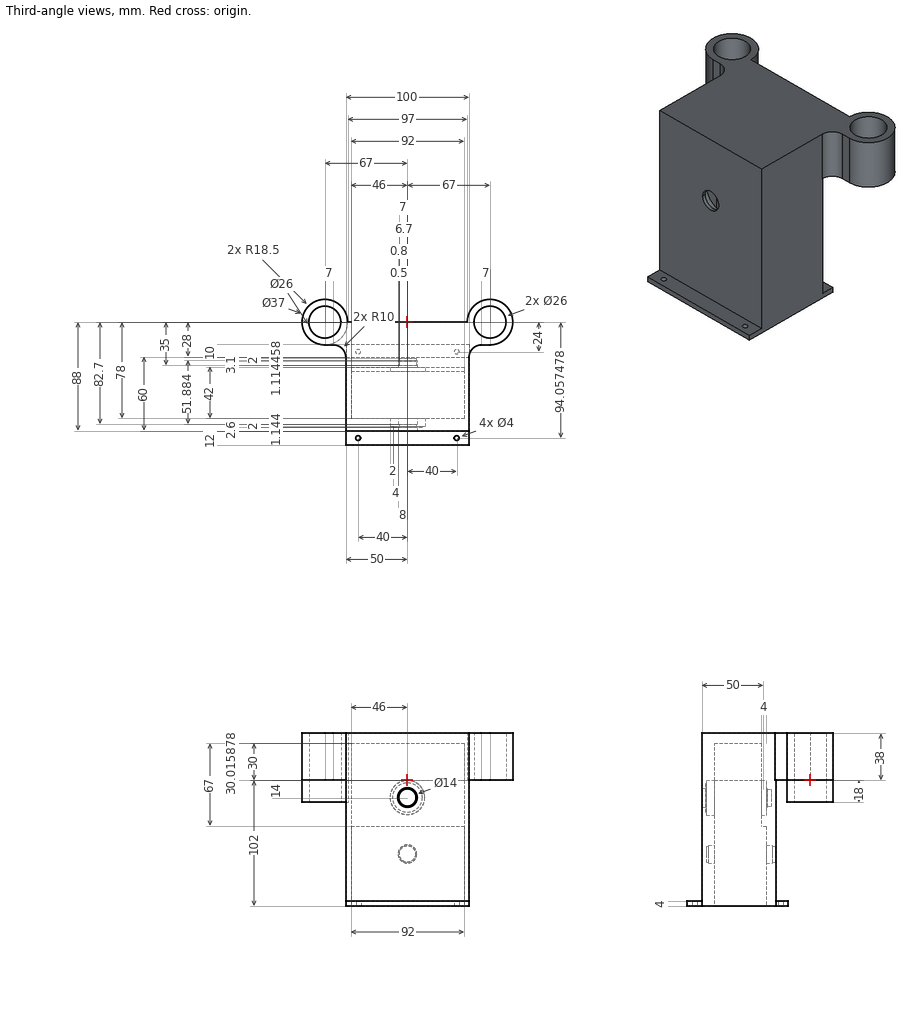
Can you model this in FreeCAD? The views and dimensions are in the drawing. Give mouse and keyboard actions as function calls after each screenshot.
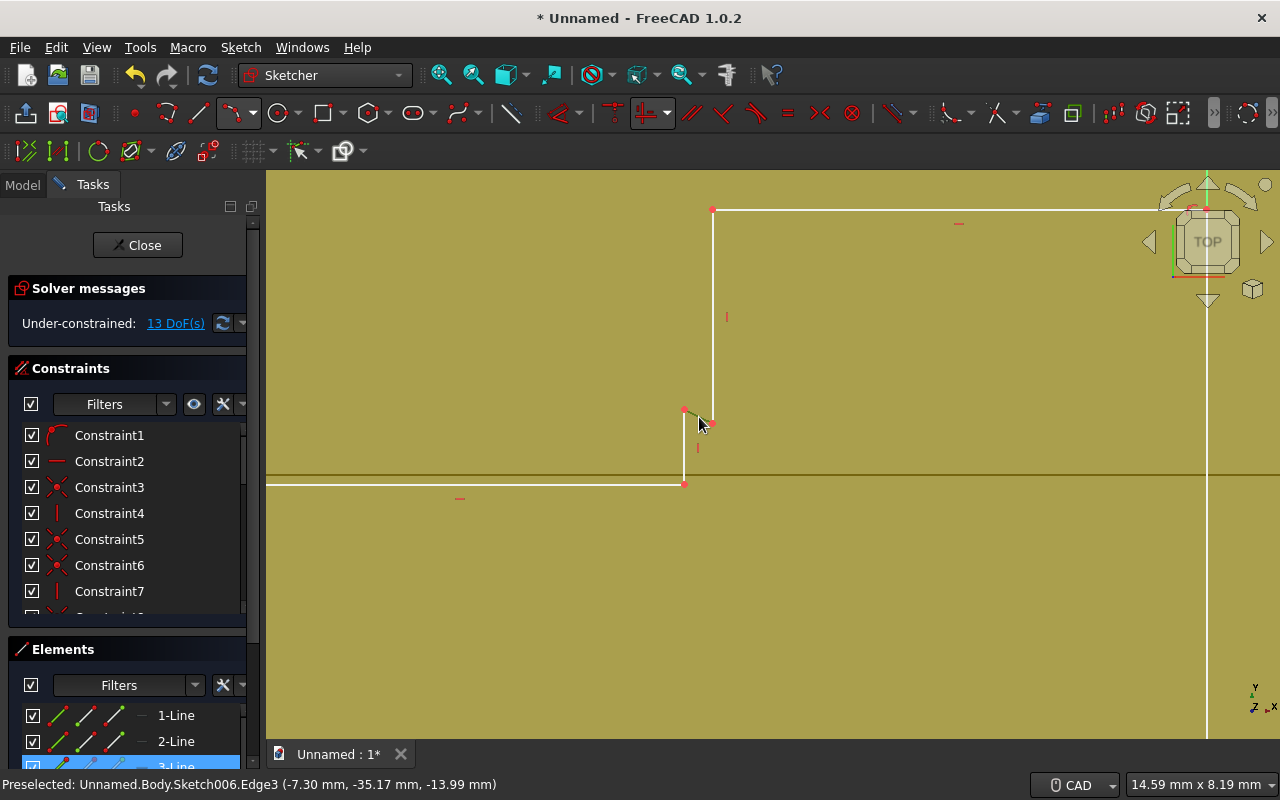
key(h)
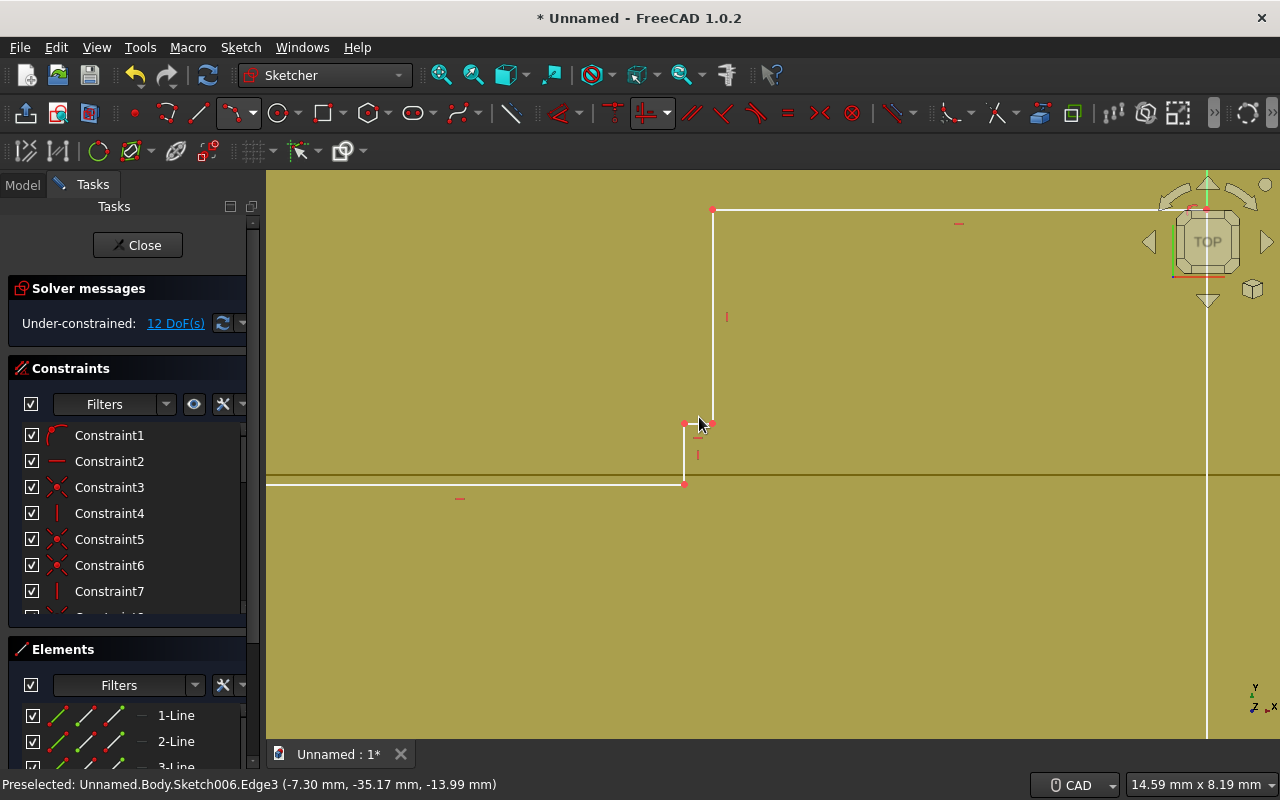
scroll(703, 417, down, 14)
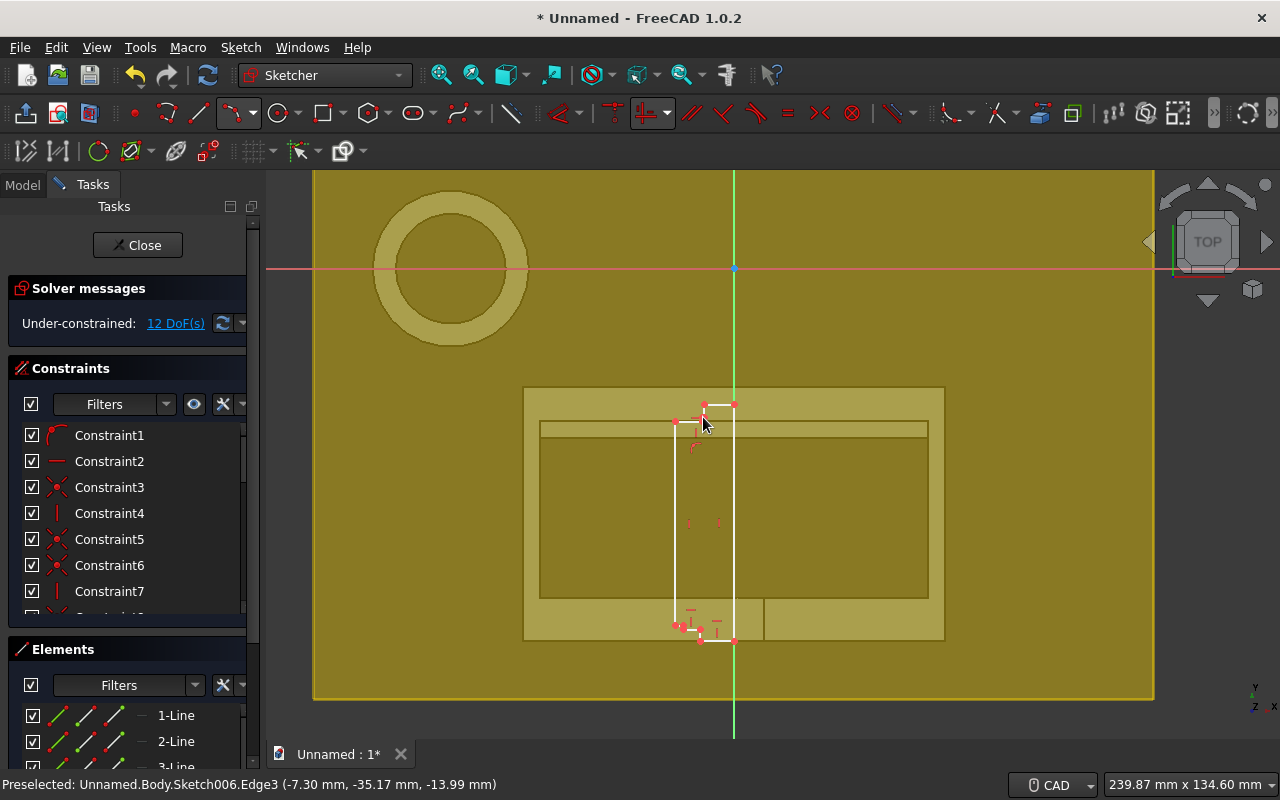
scroll(677, 626, up, 9)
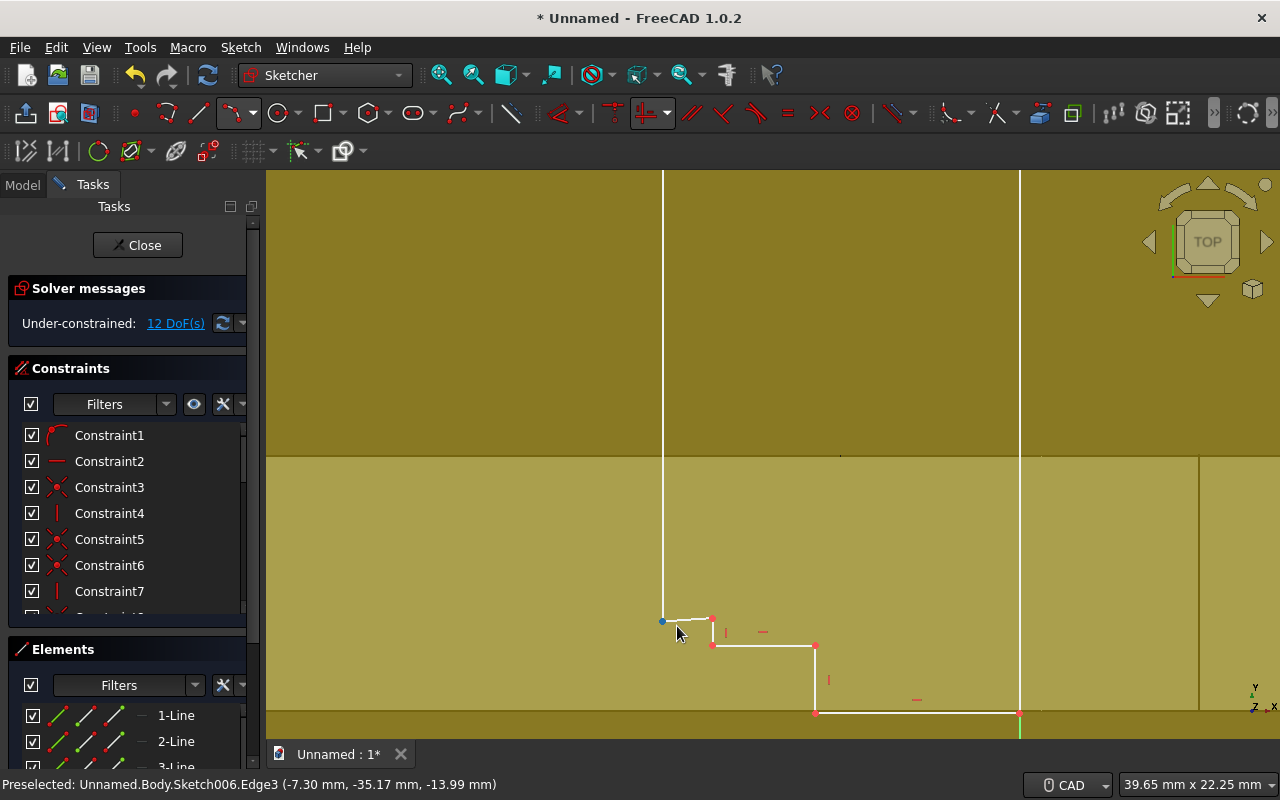
click(678, 620)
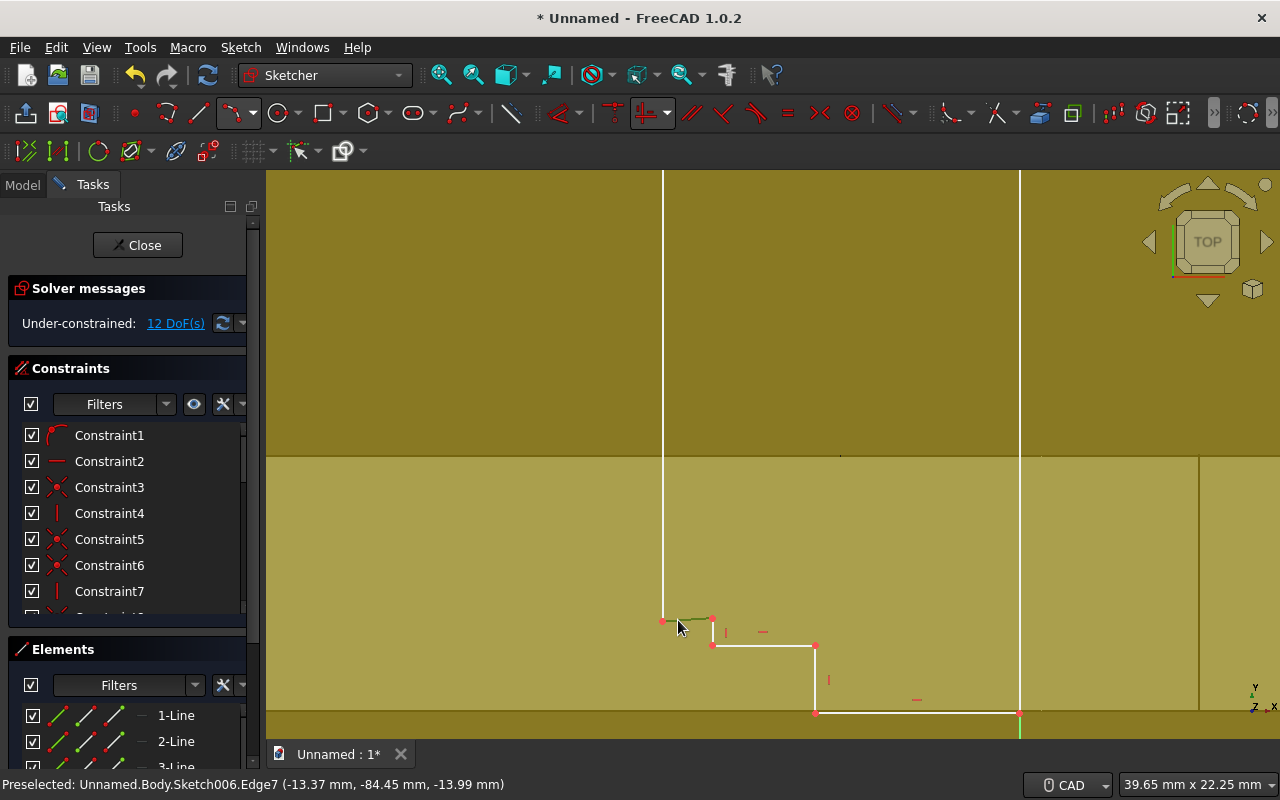
click(670, 114)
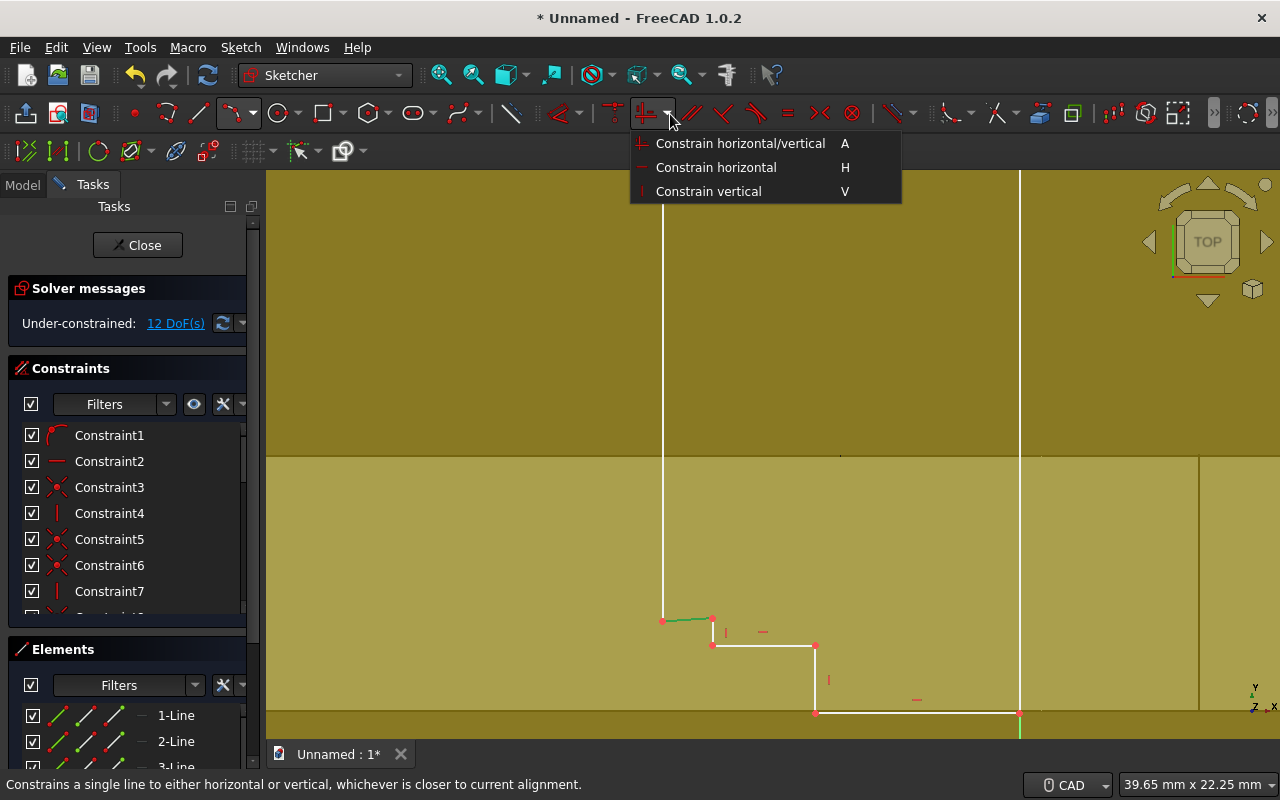
click(766, 167)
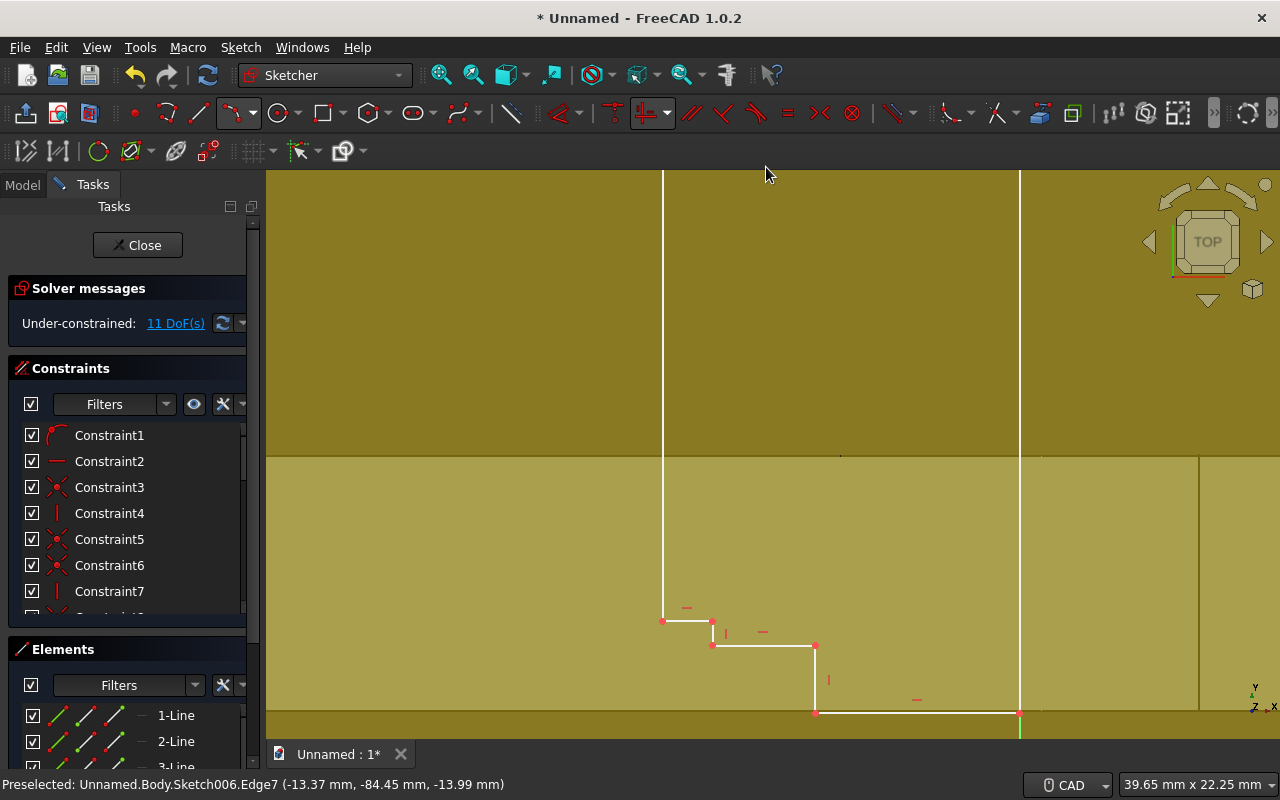
key(d)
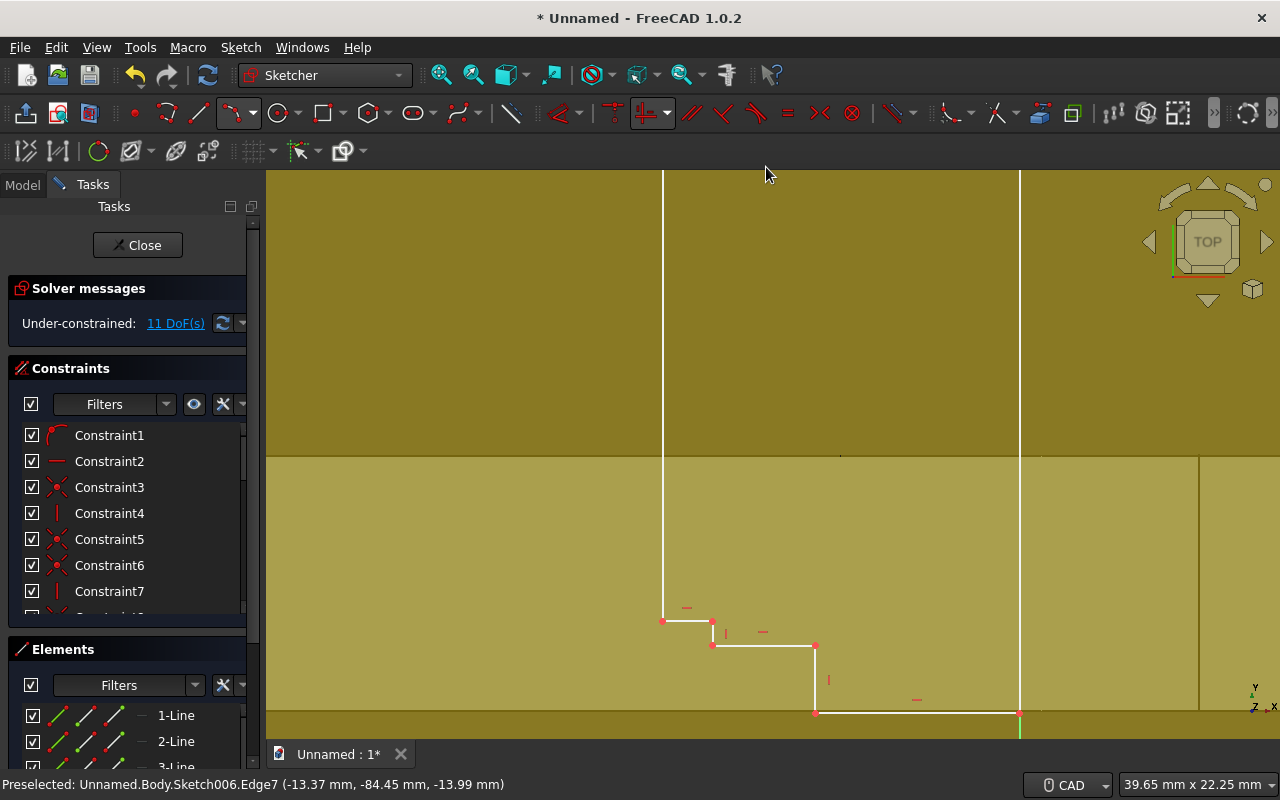
scroll(677, 626, down, 9)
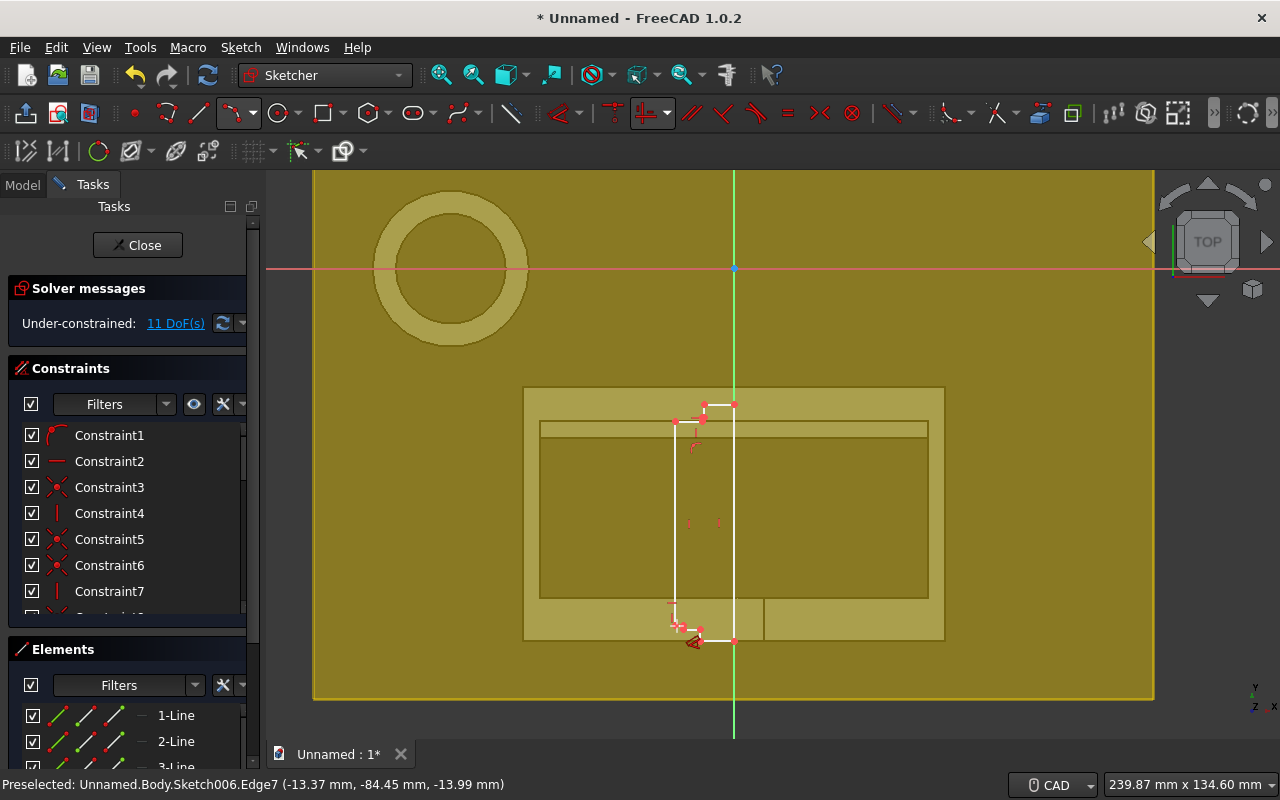
scroll(725, 405, up, 3)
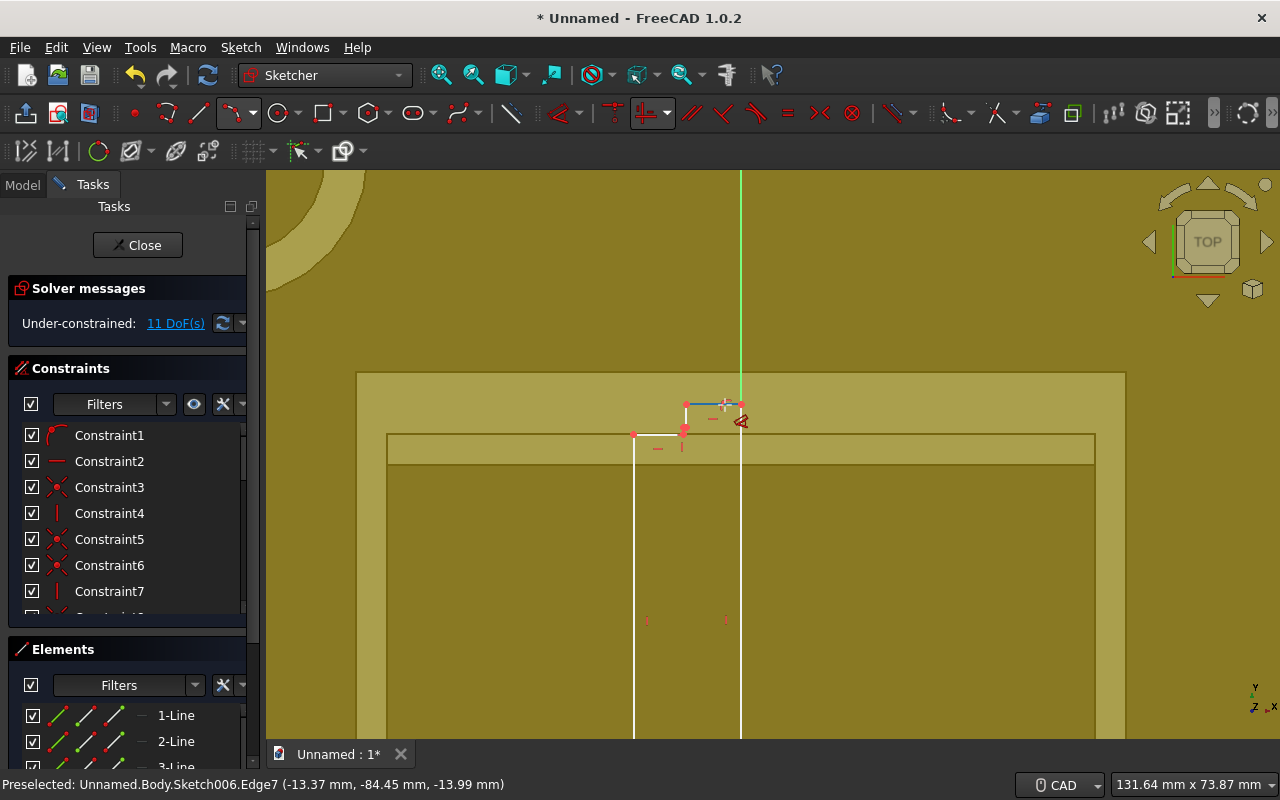
click(725, 404)
click(714, 370)